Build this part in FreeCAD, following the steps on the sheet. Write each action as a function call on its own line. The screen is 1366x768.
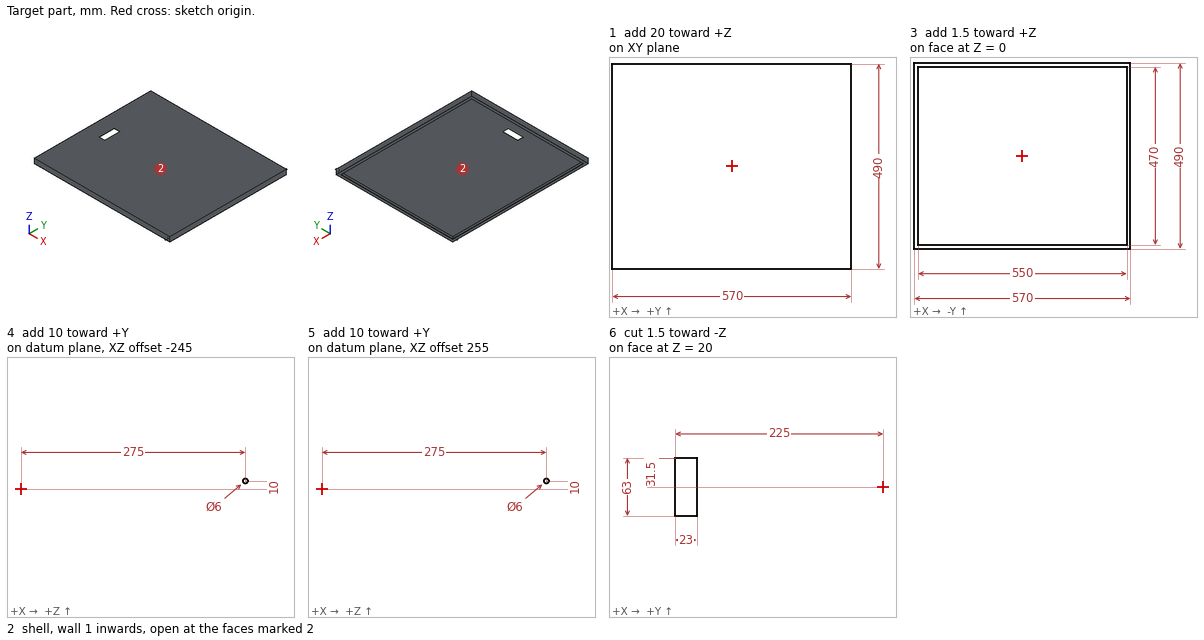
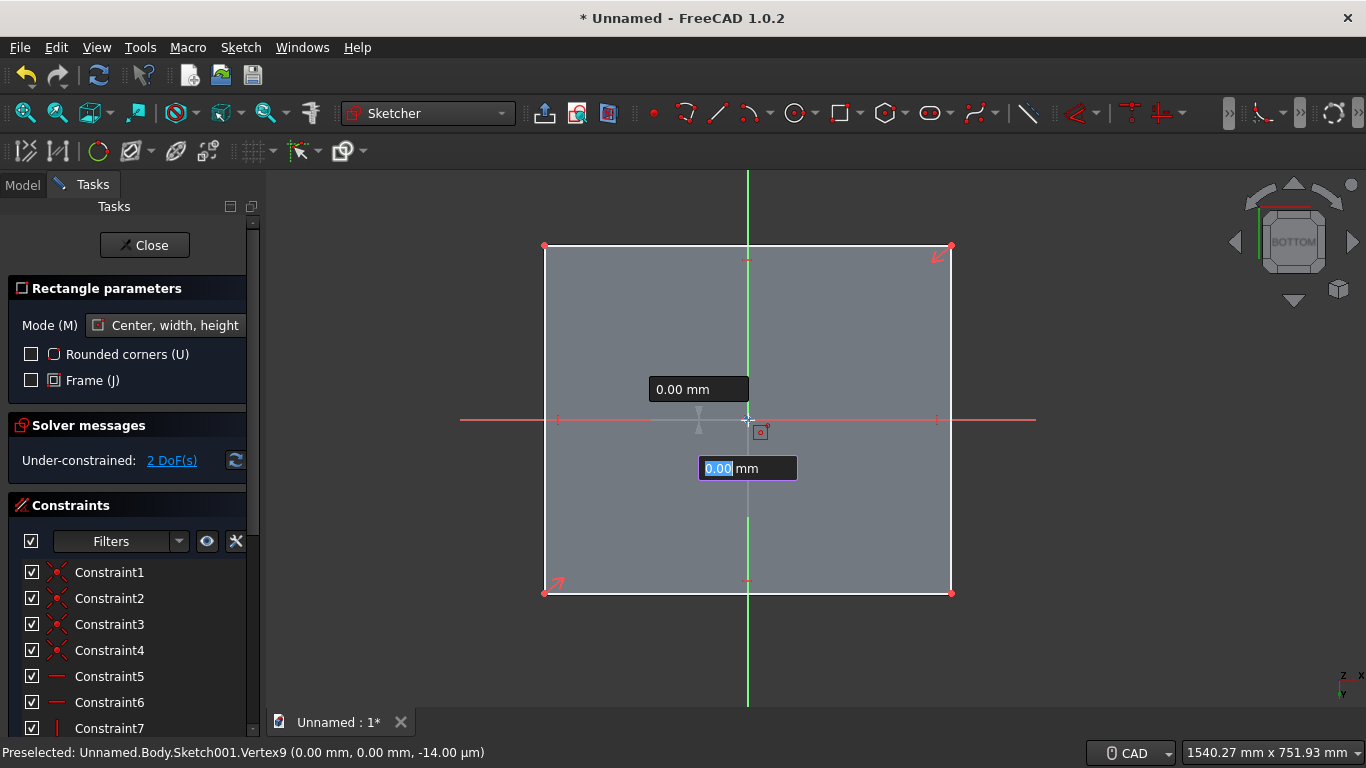
scroll(944, 252, up, 4)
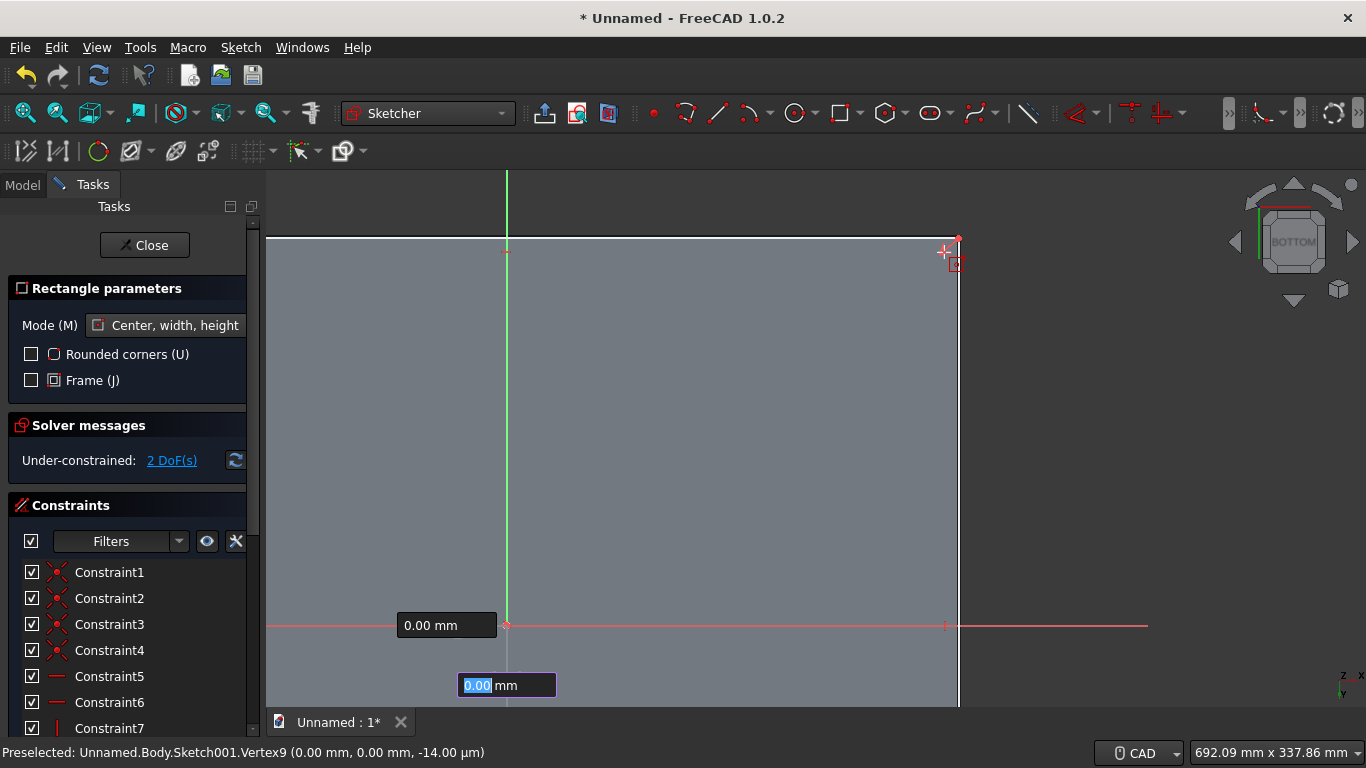
click(944, 252)
key(Escape)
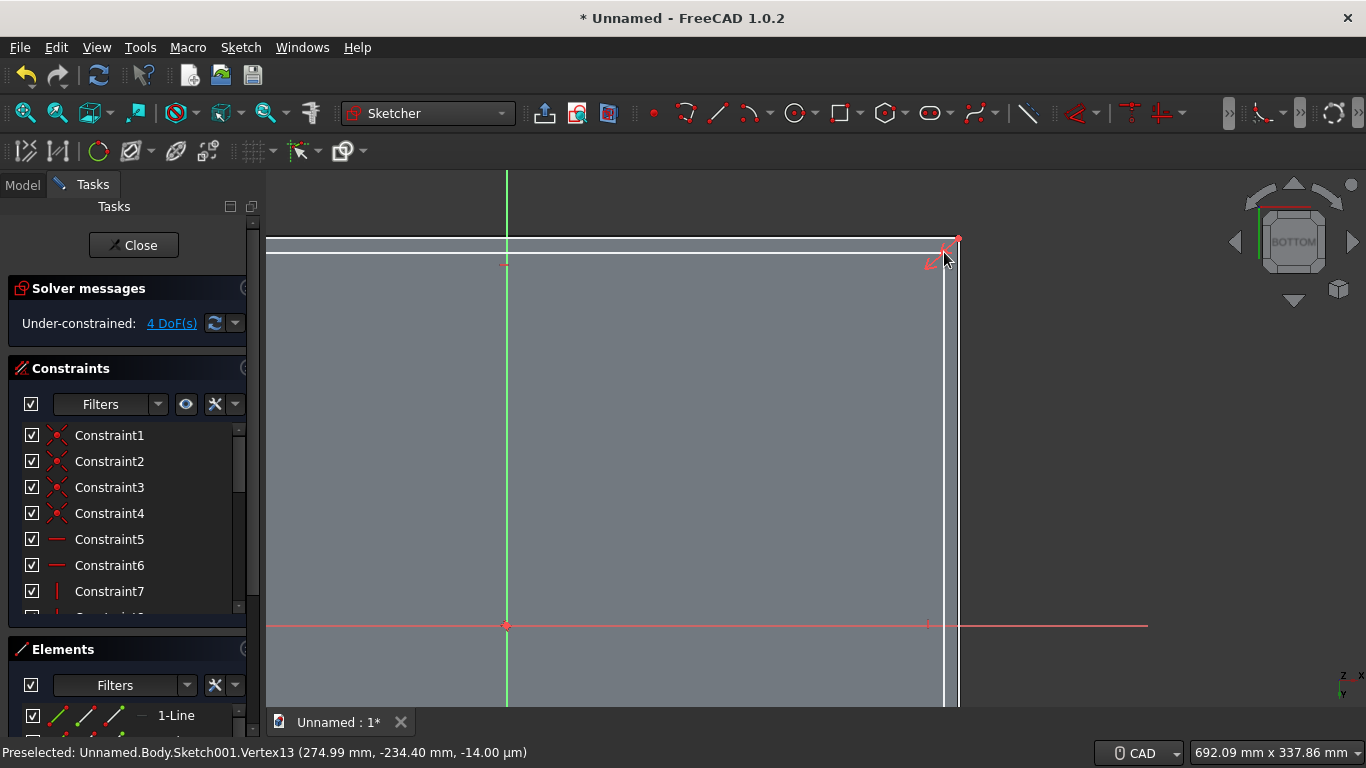
scroll(944, 286, down, 4)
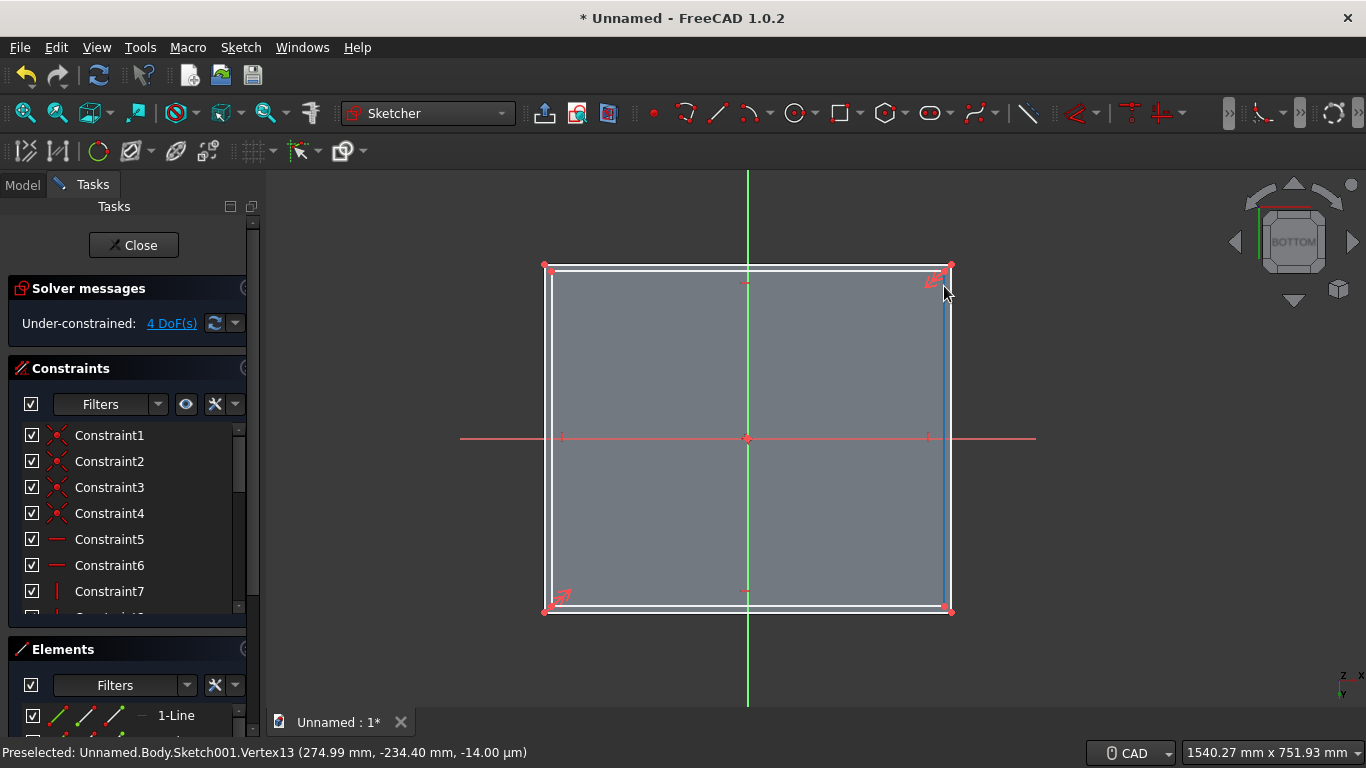
scroll(667, 613, up, 4)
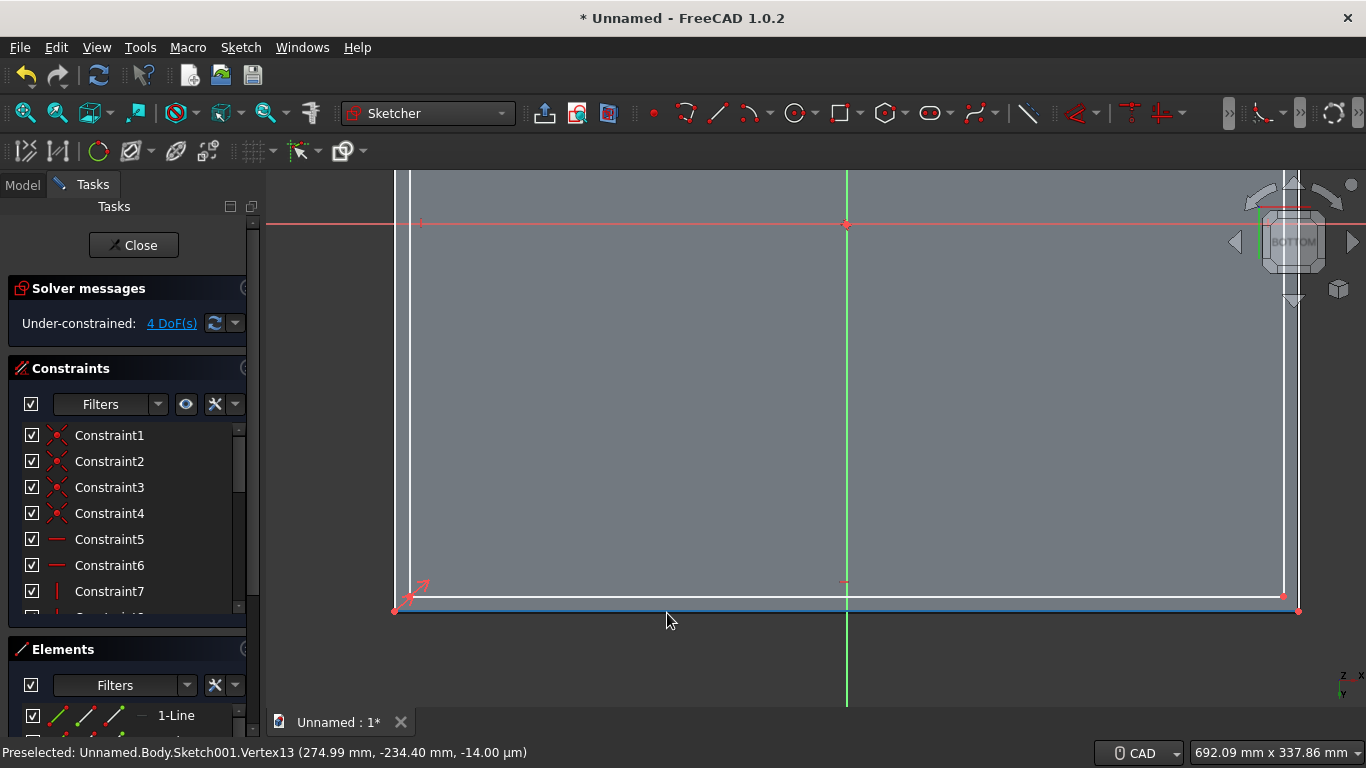
click(666, 611)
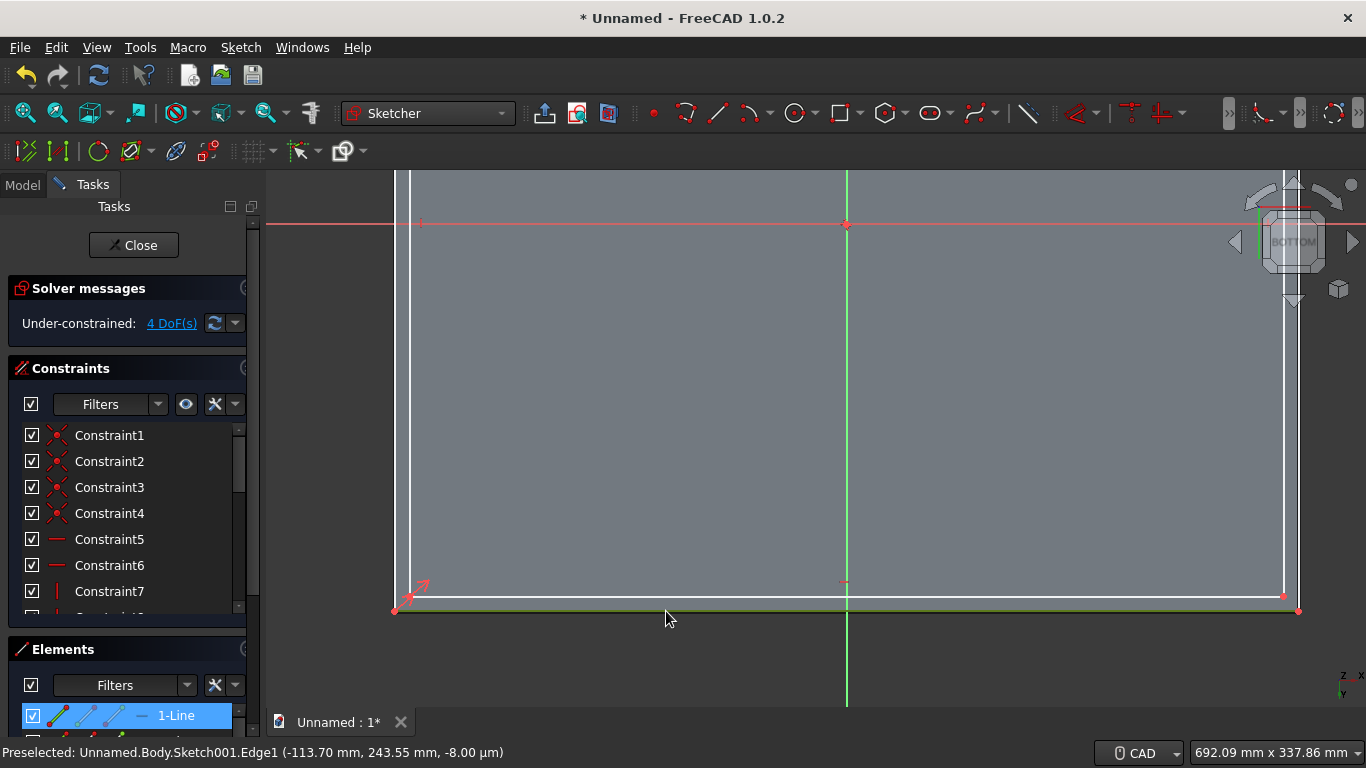
key(l)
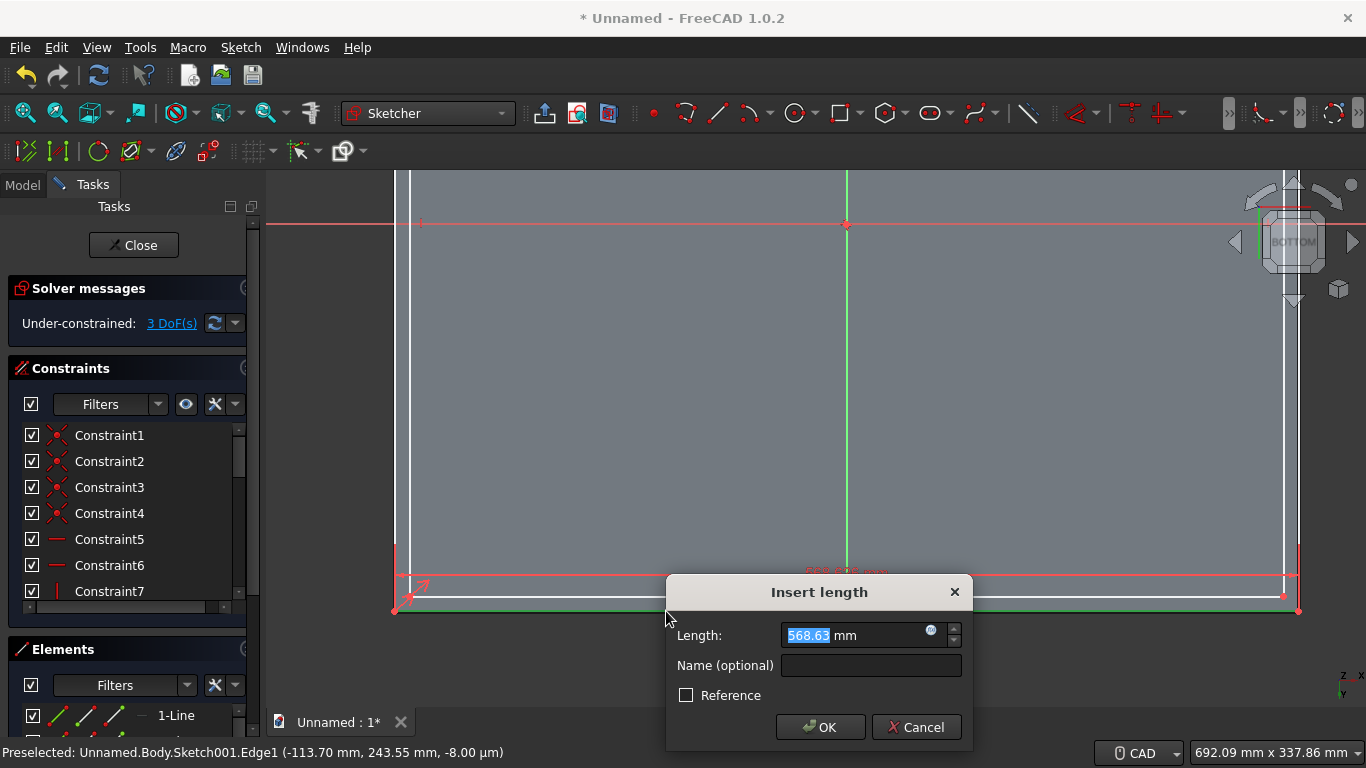
text(570)
key(Return)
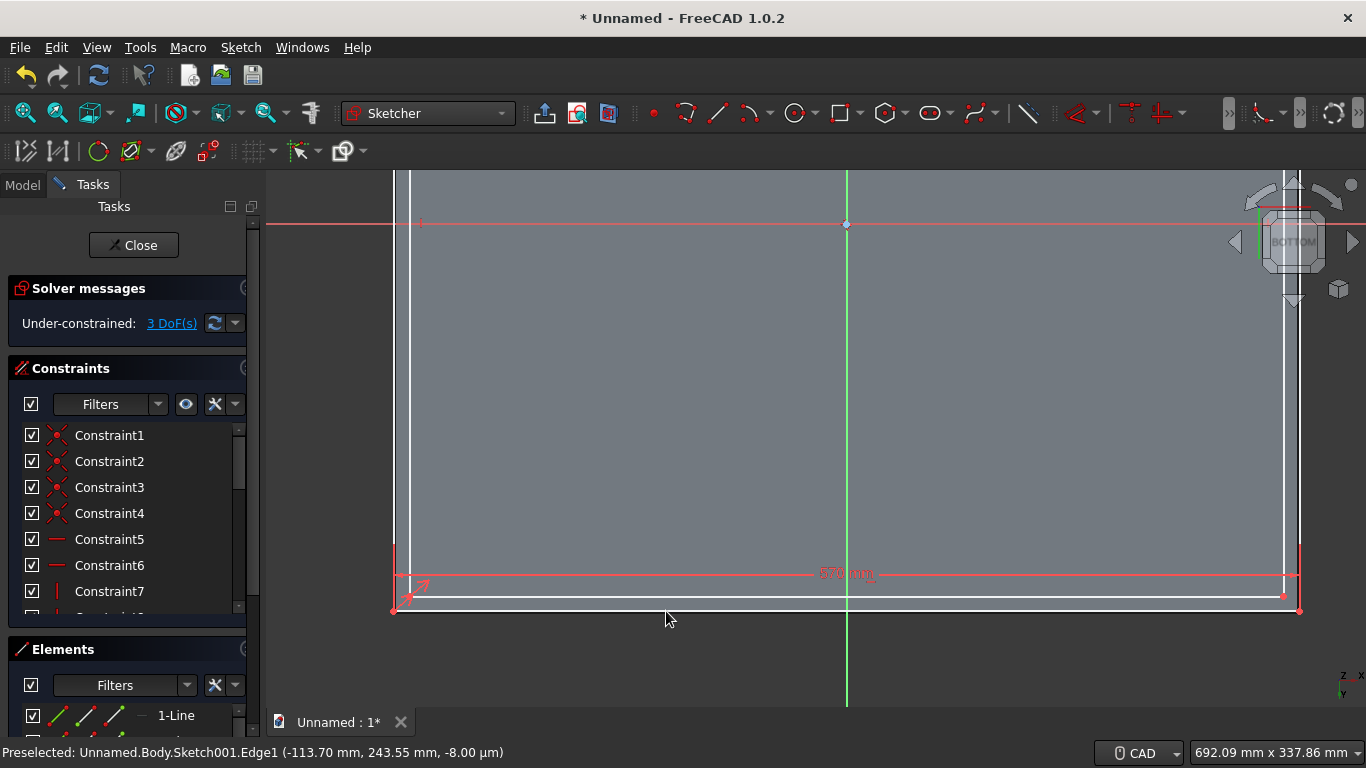
scroll(667, 613, down, 4)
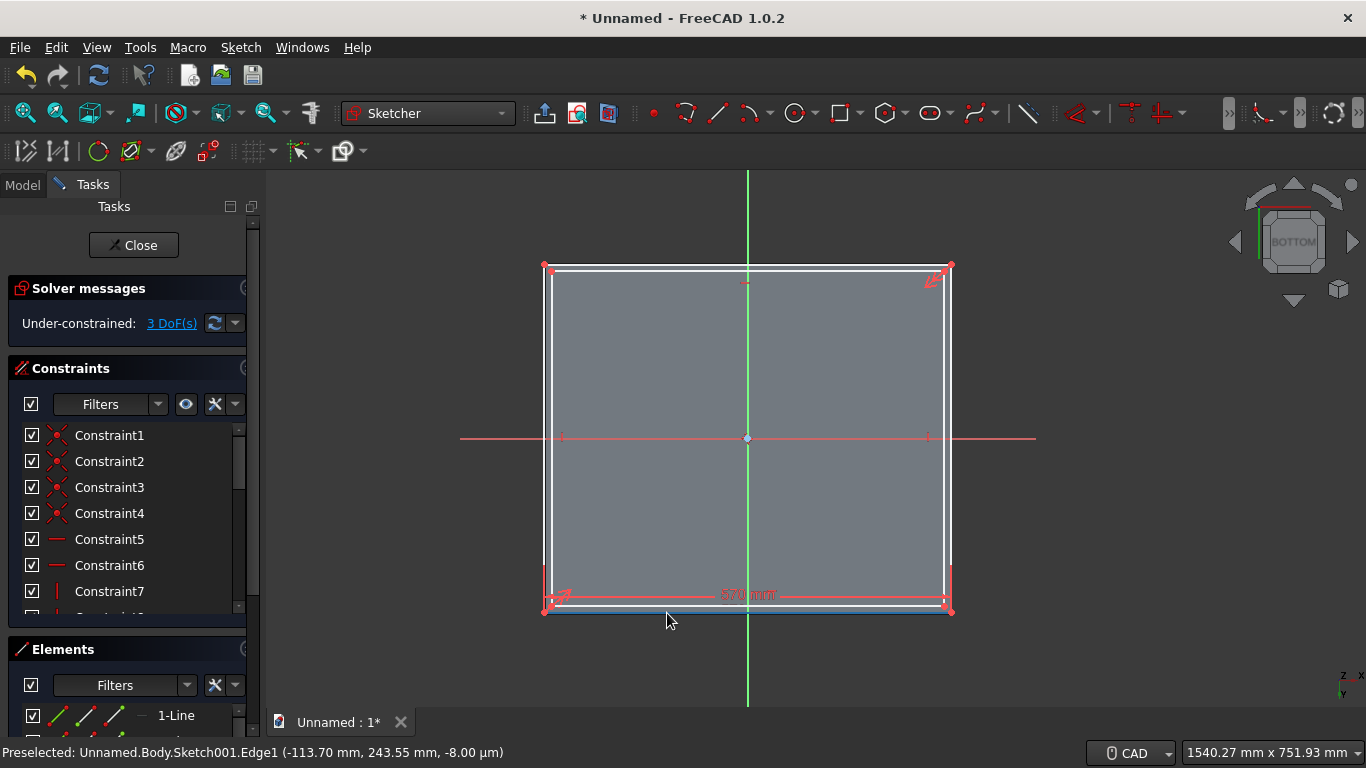
scroll(951, 508, up, 4)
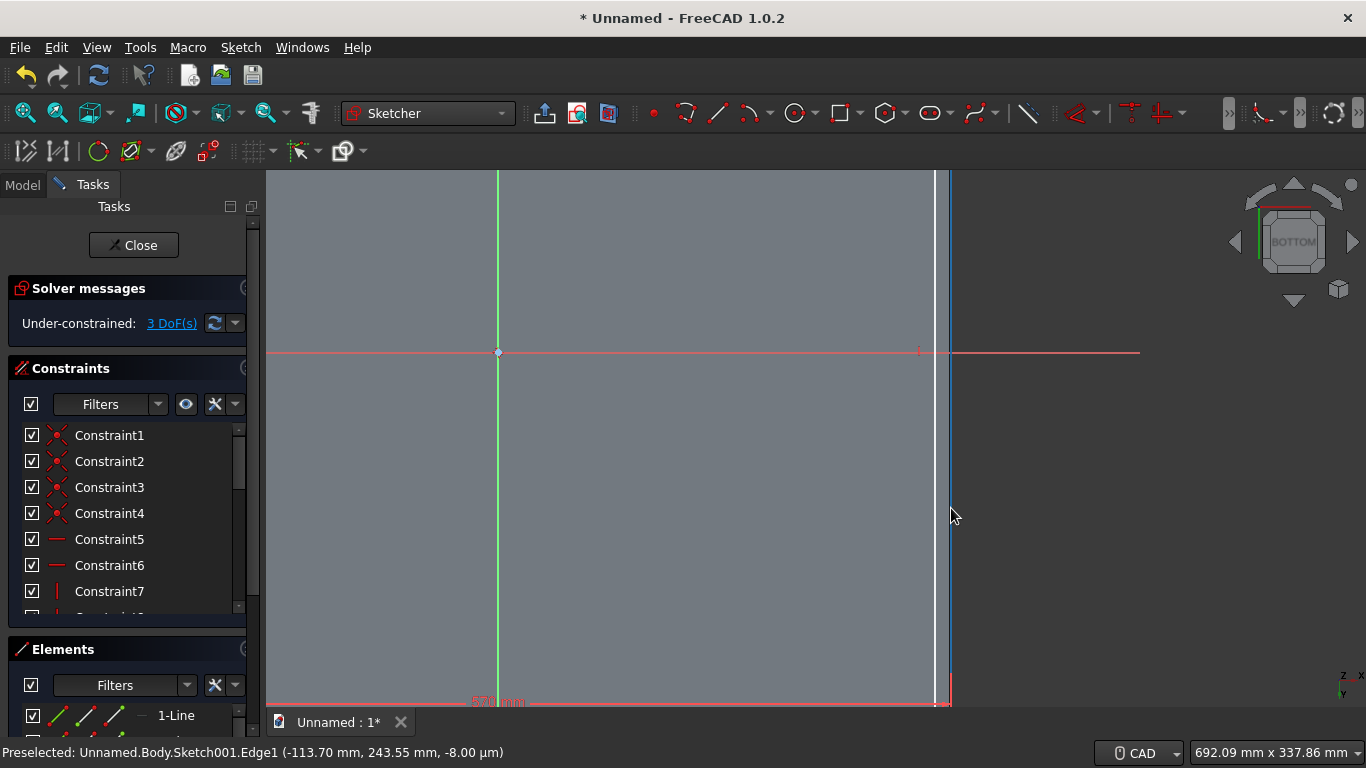
click(951, 508)